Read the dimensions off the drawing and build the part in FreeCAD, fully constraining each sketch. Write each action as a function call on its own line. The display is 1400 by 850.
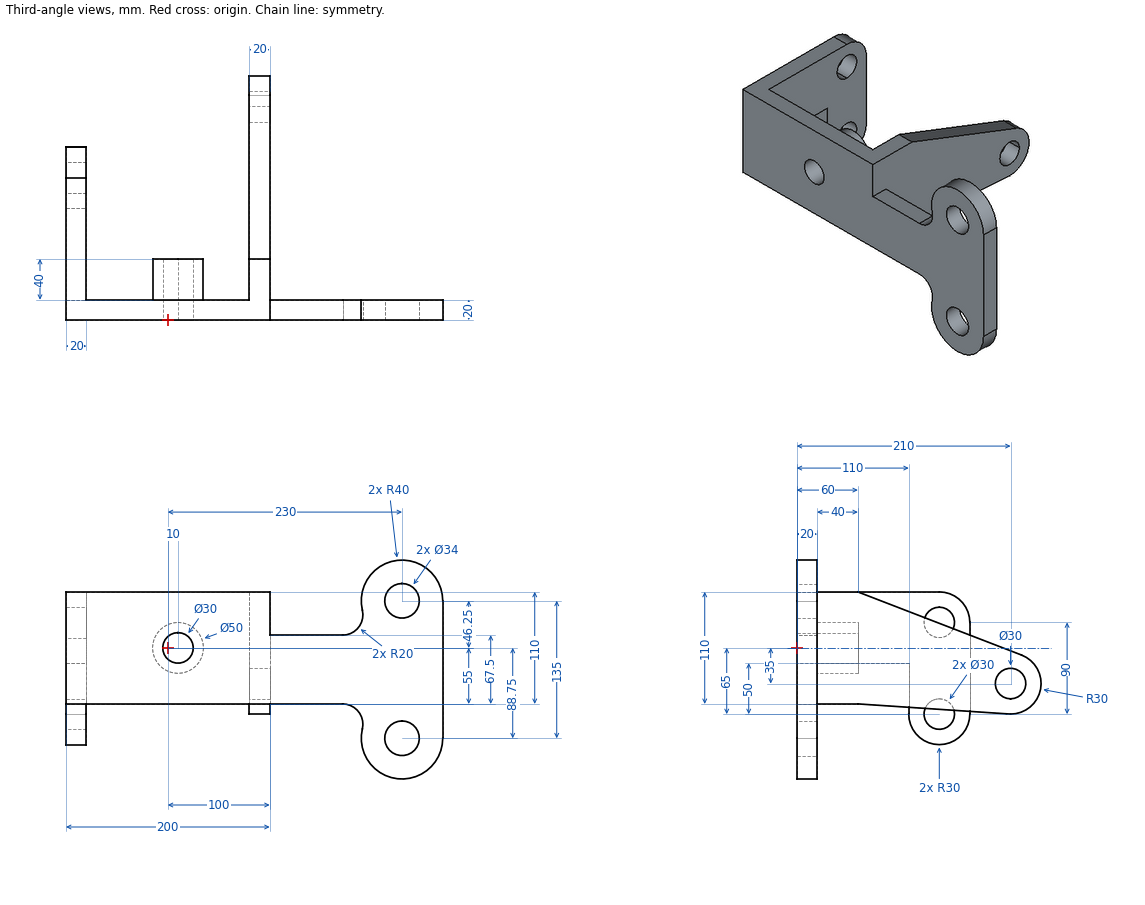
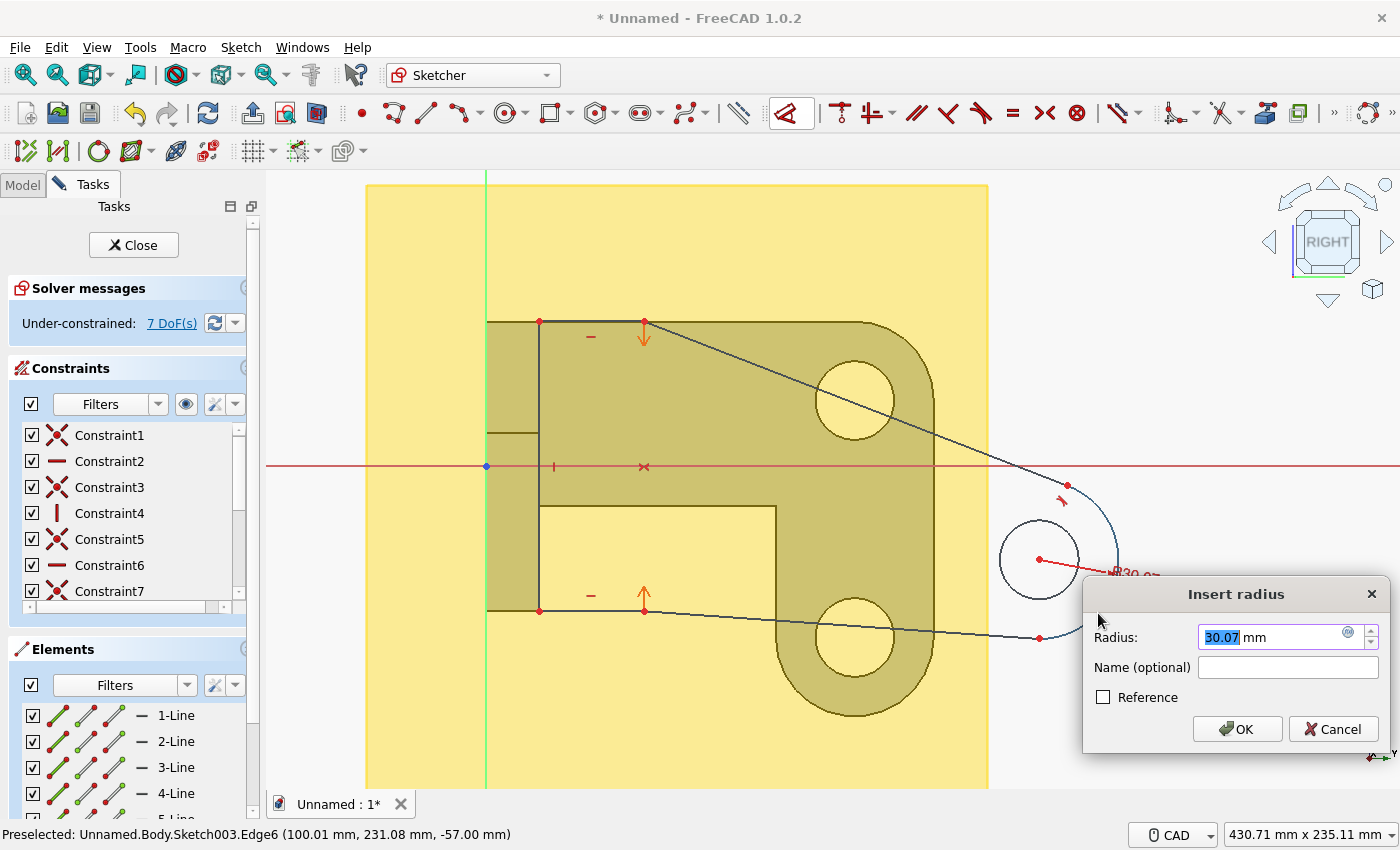
text(30)
key(Return)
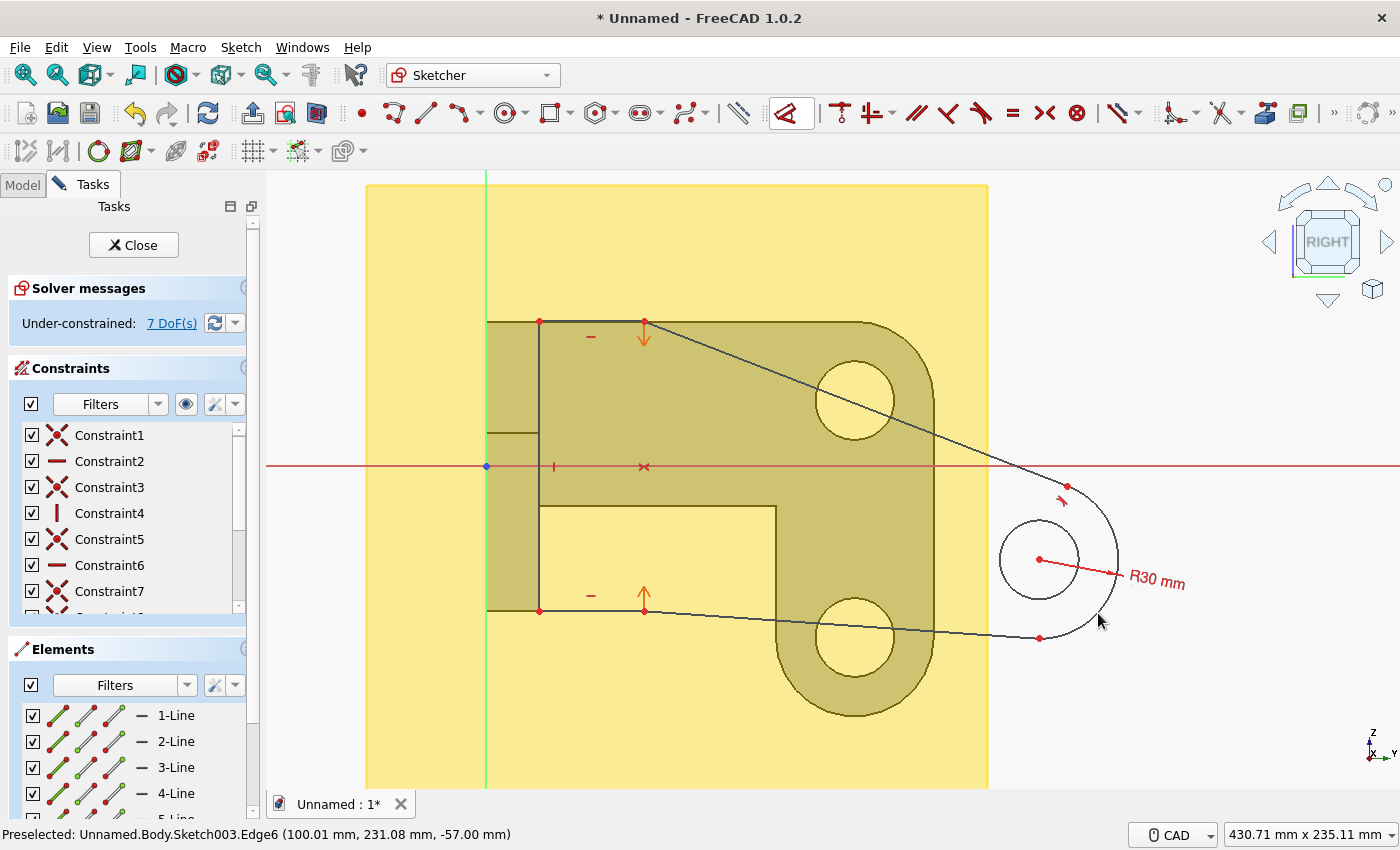
click(1067, 532)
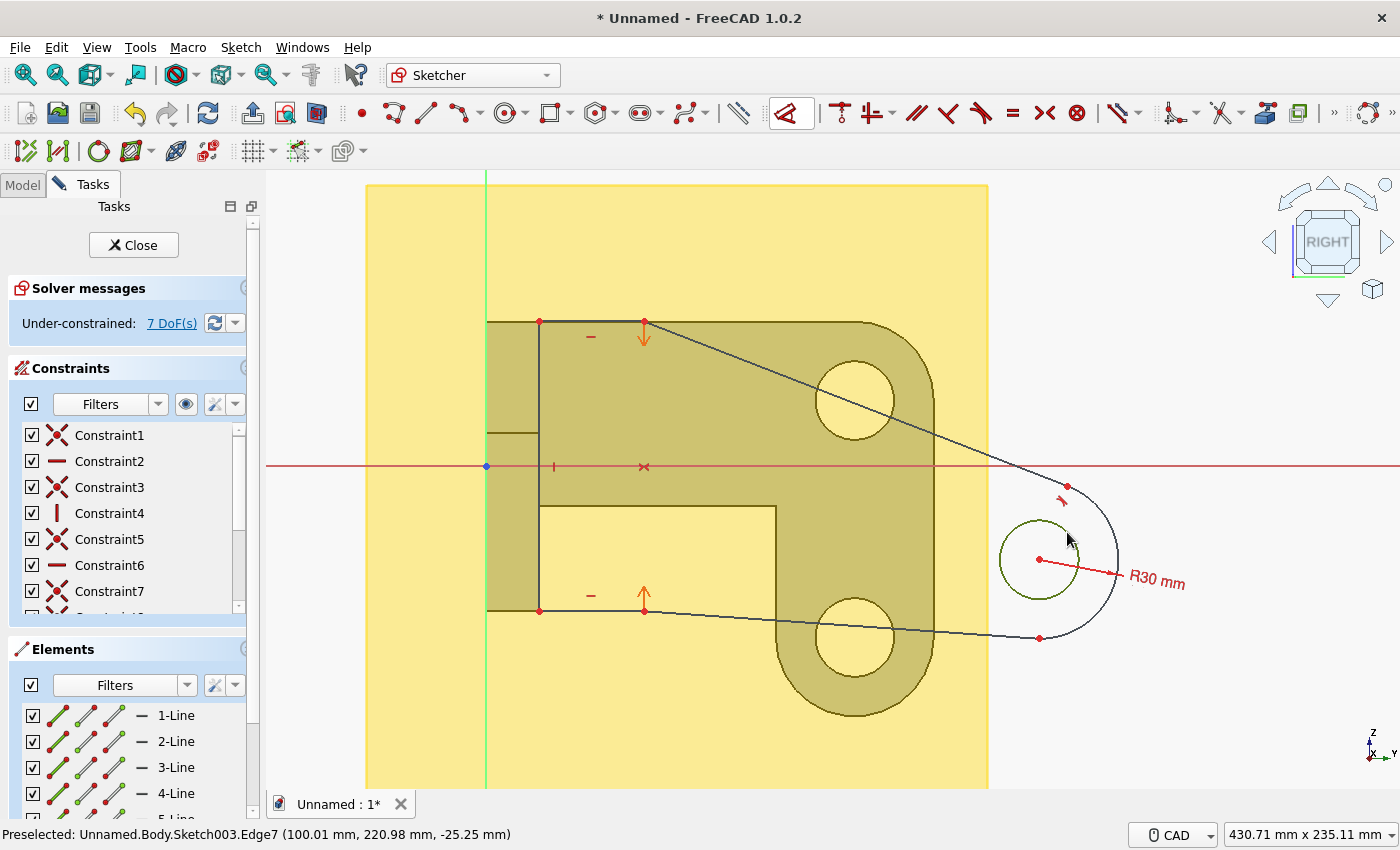
key(k)
key(o)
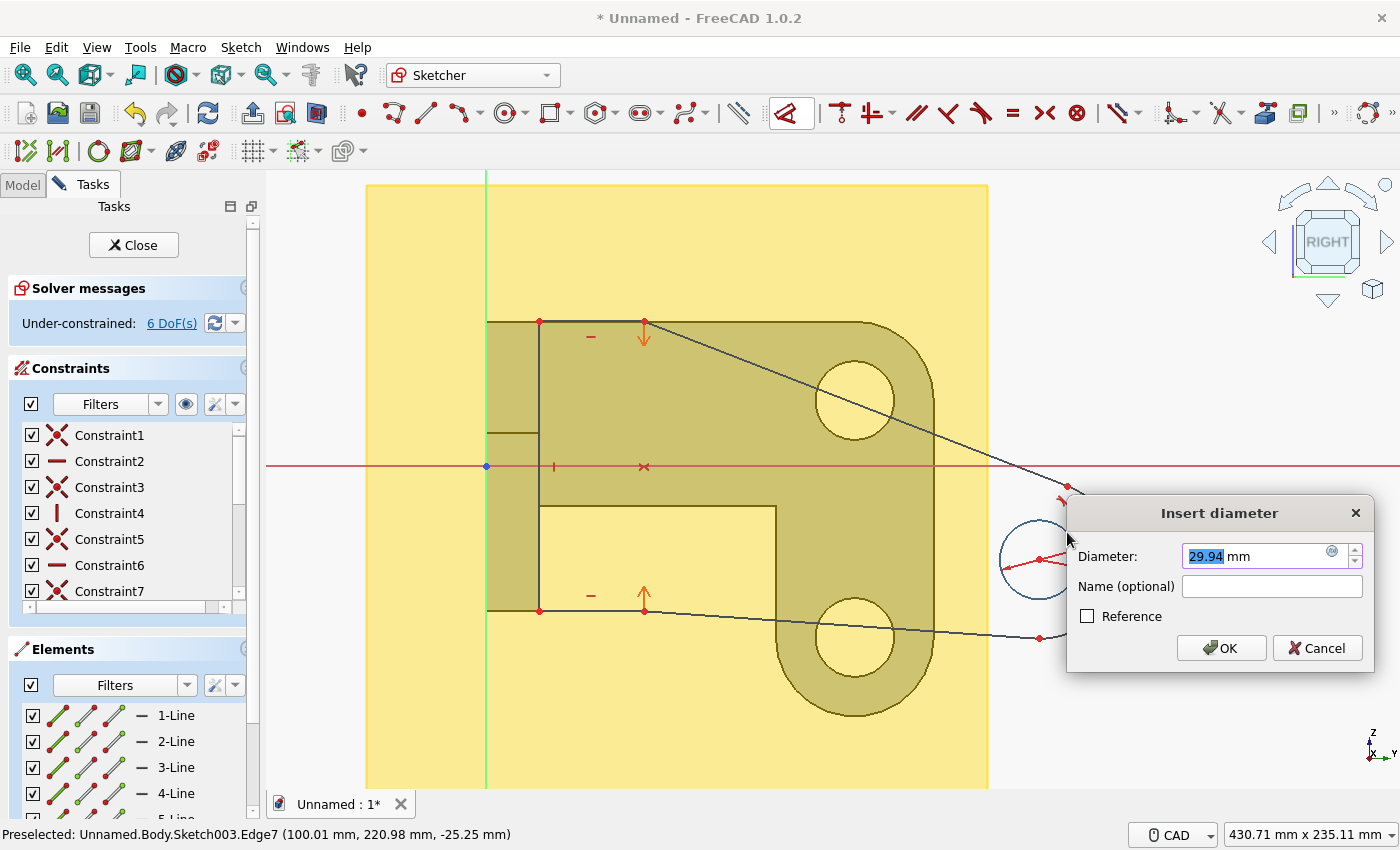
text(30)
key(Return)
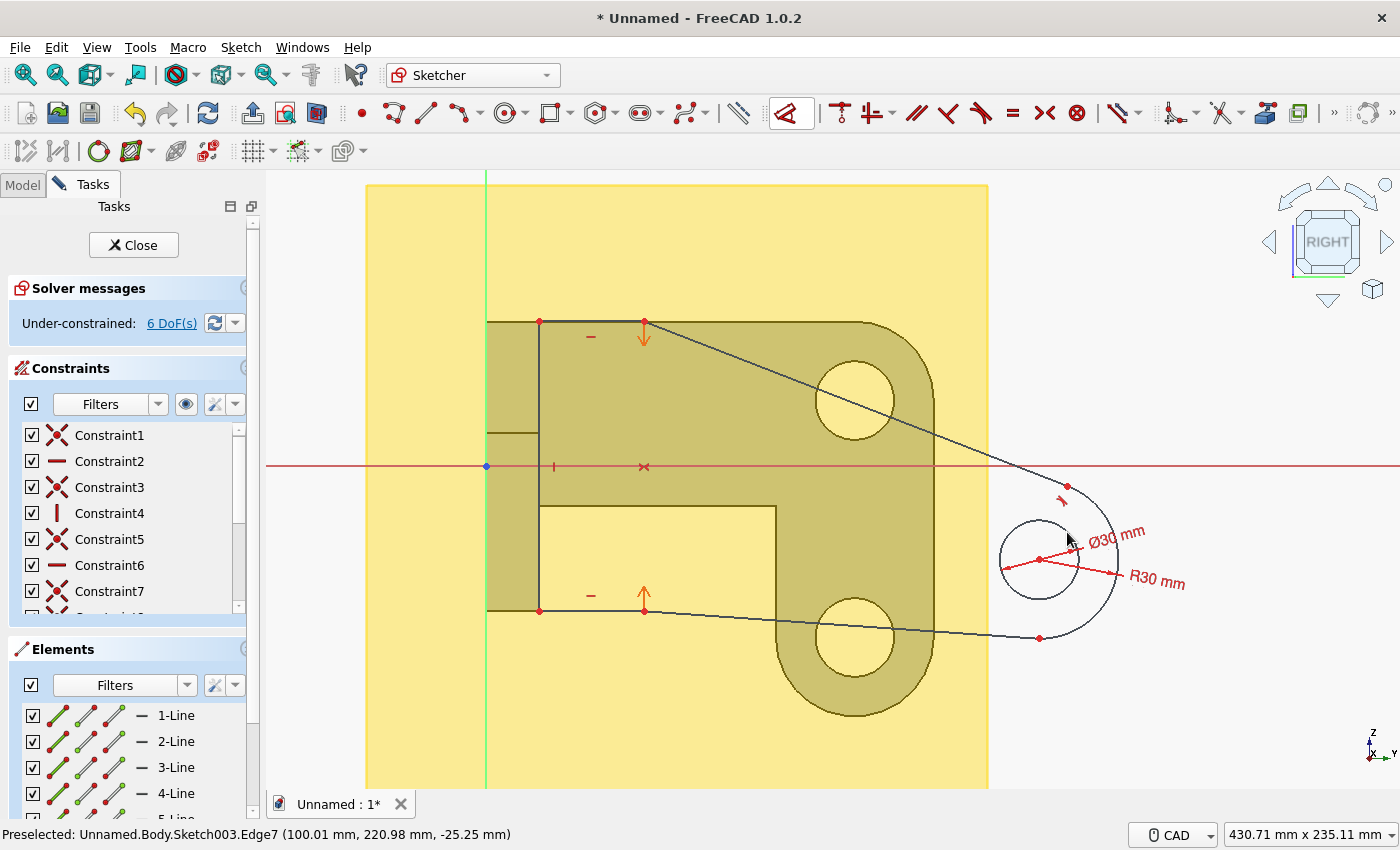
click(613, 321)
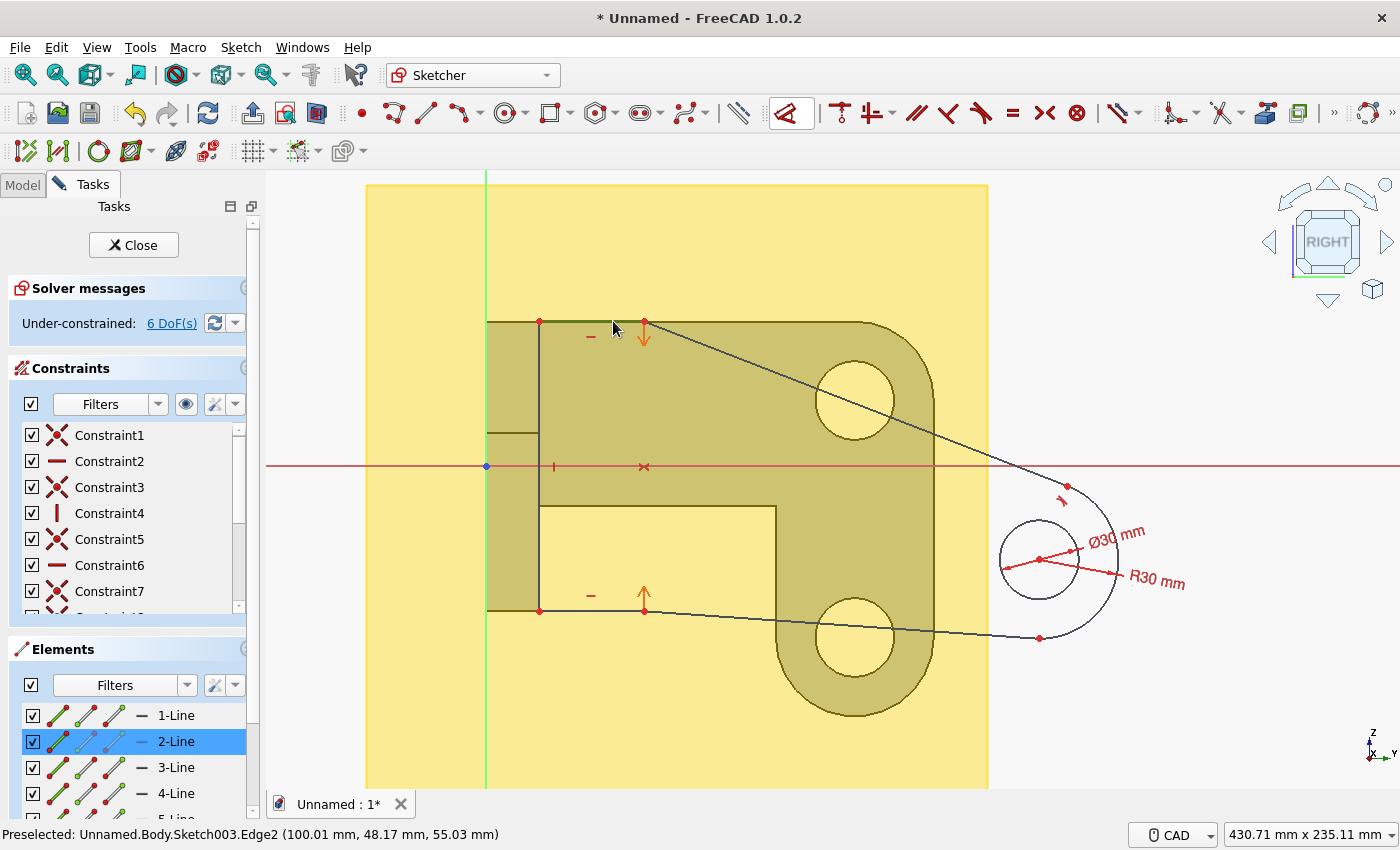
key(l)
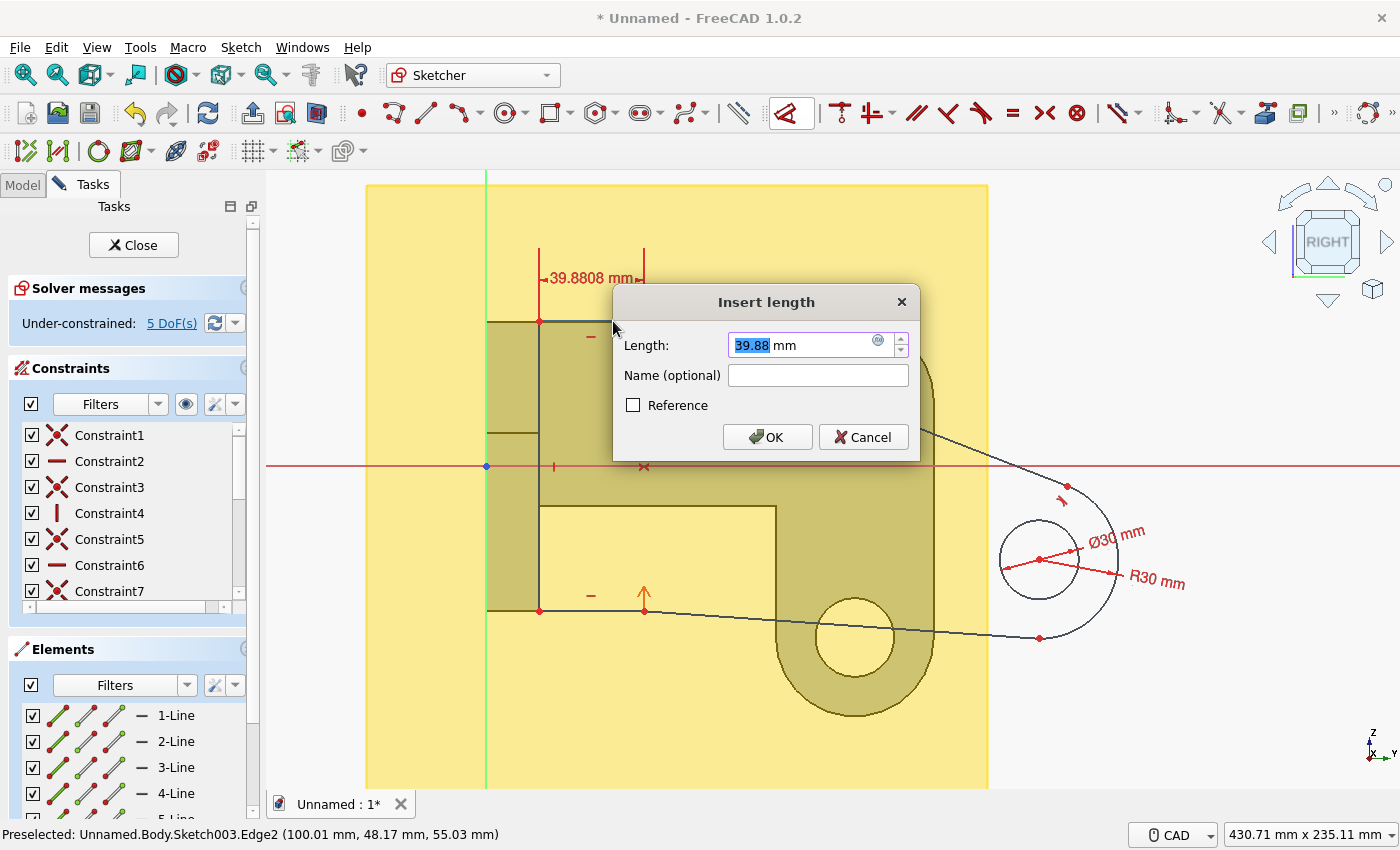
text(40)
key(Return)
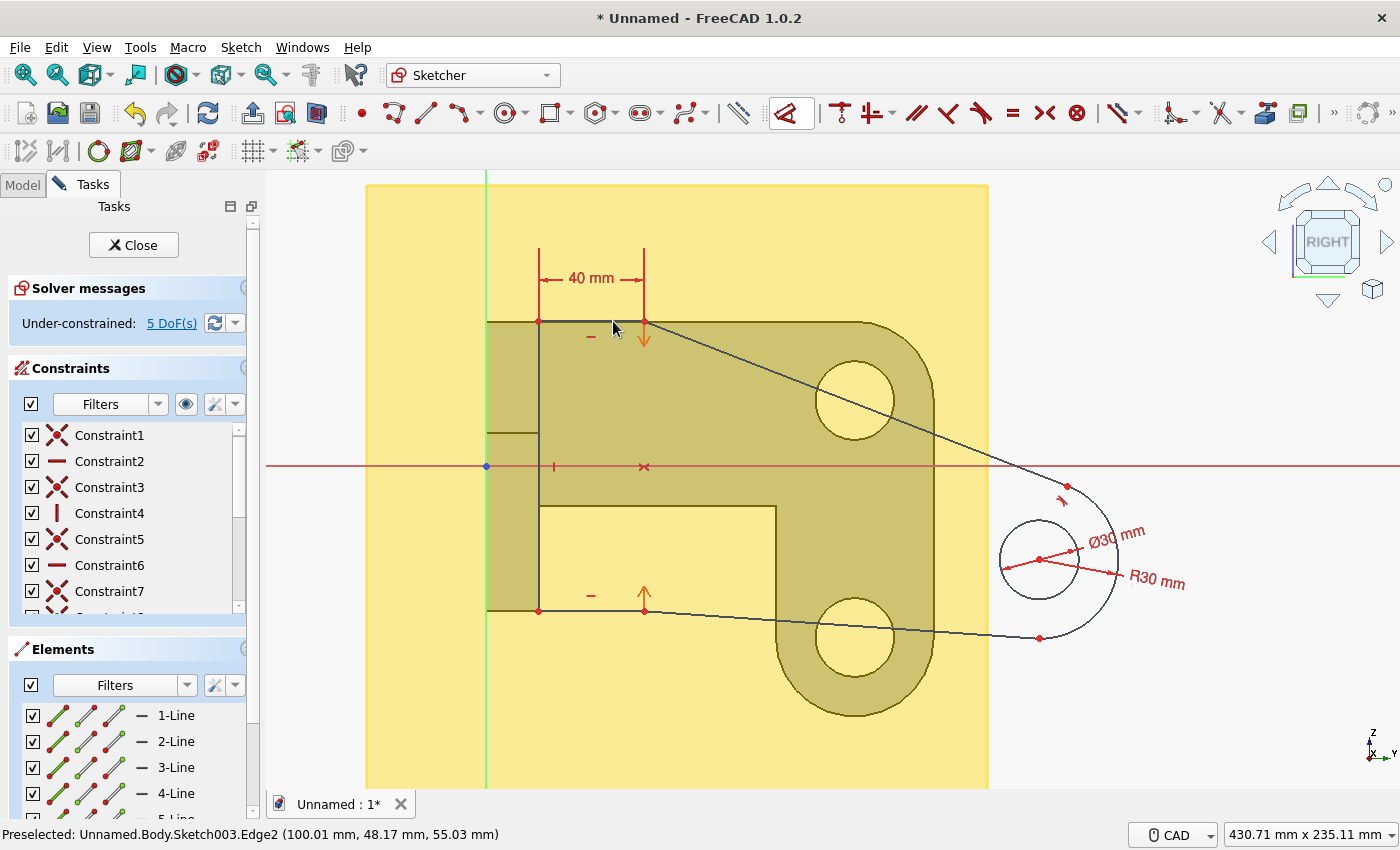
click(1039, 560)